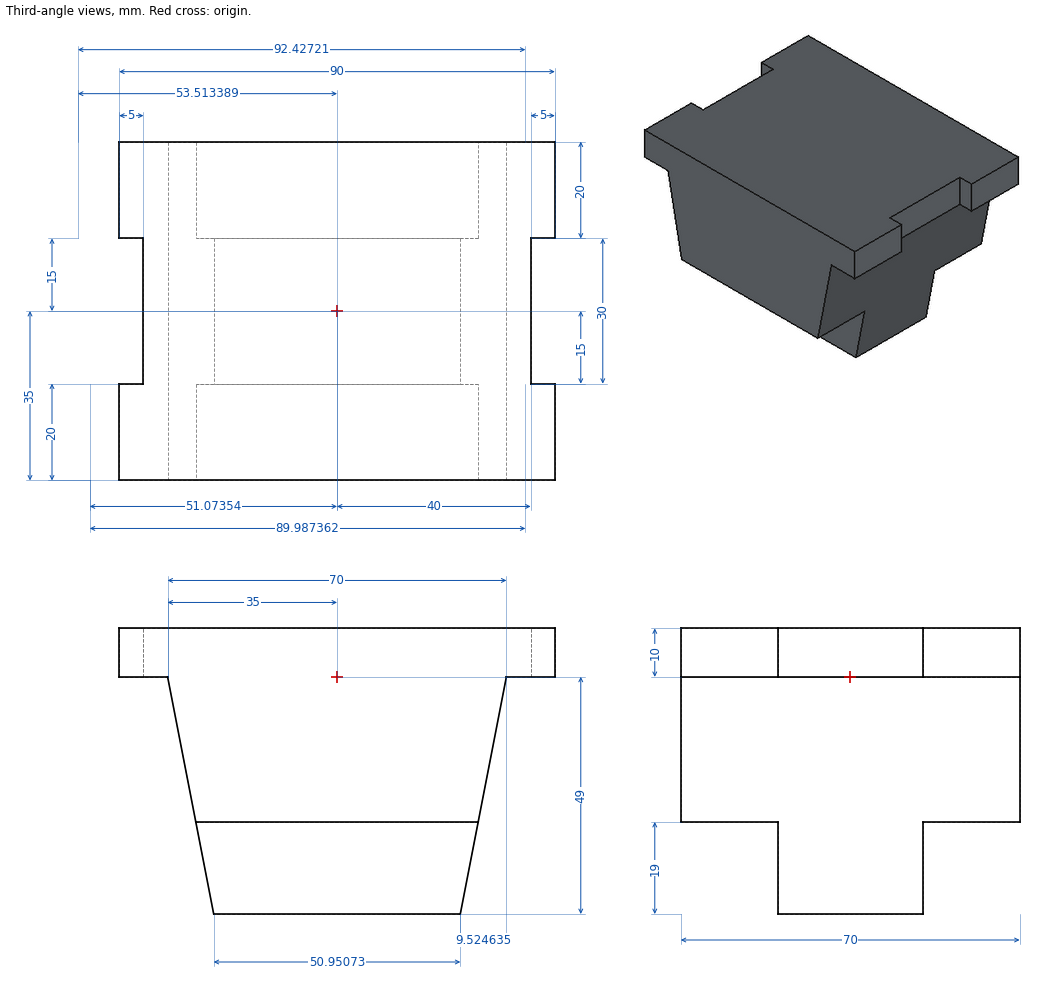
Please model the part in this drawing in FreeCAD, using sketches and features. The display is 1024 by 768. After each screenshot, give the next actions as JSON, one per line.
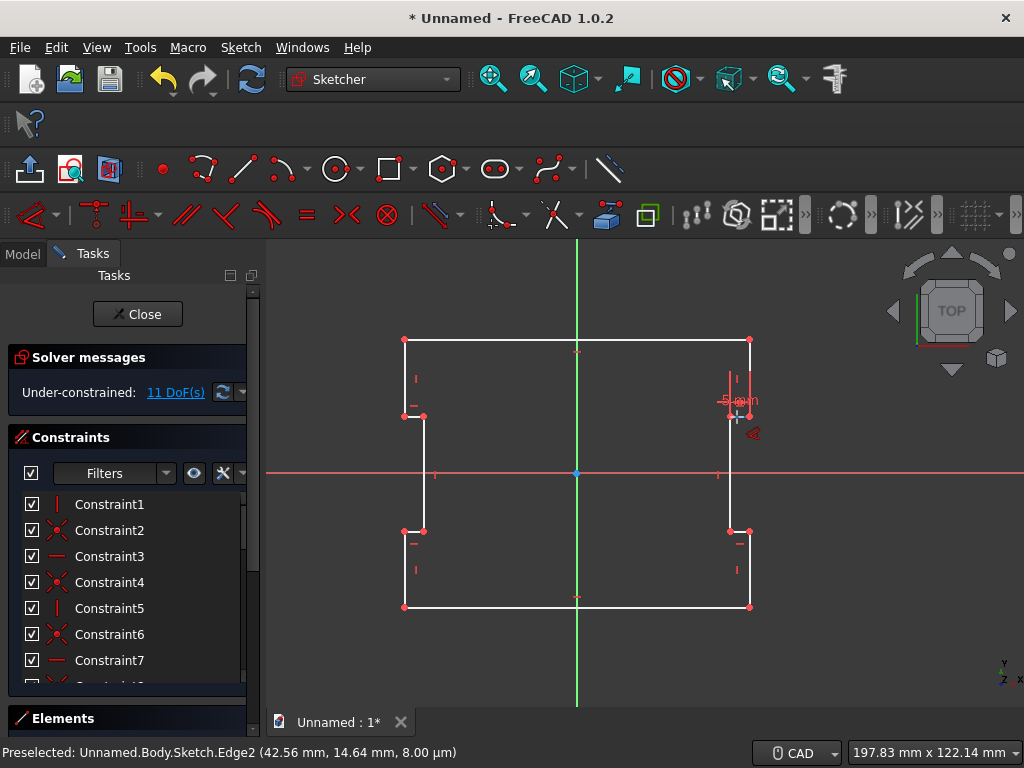
{"action": "scroll", "coordinate": [410, 417], "scroll_direction": "up", "scroll_amount": 5}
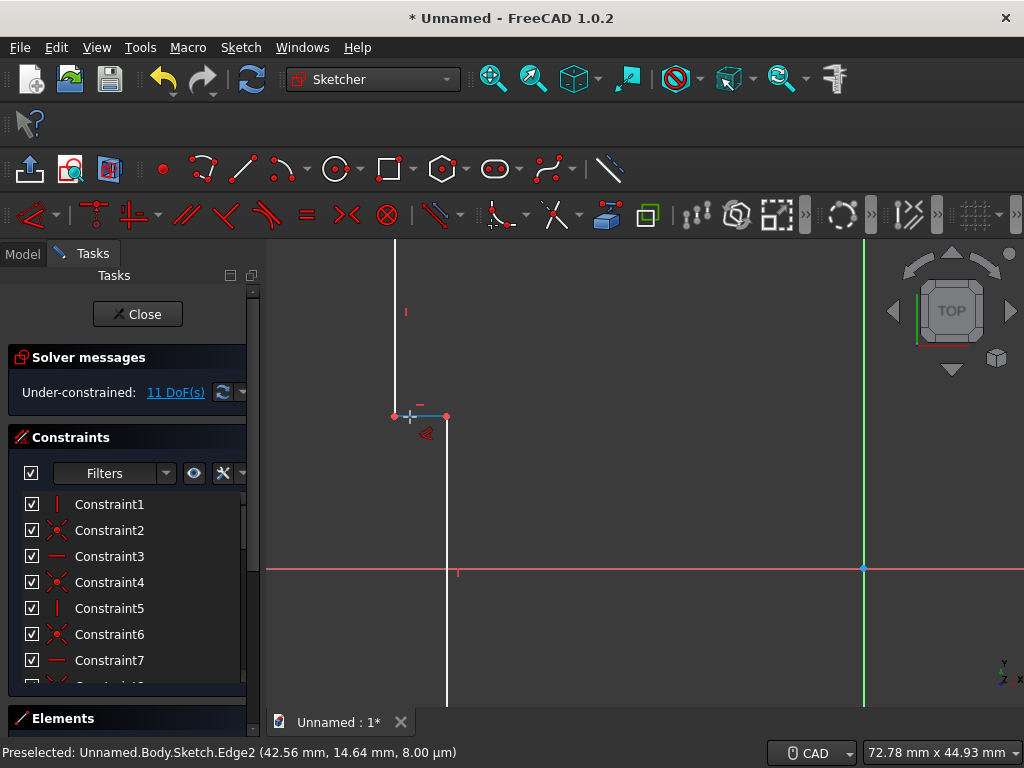
{"action": "left_click", "coordinate": [410, 416]}
{"action": "left_click", "coordinate": [421, 382]}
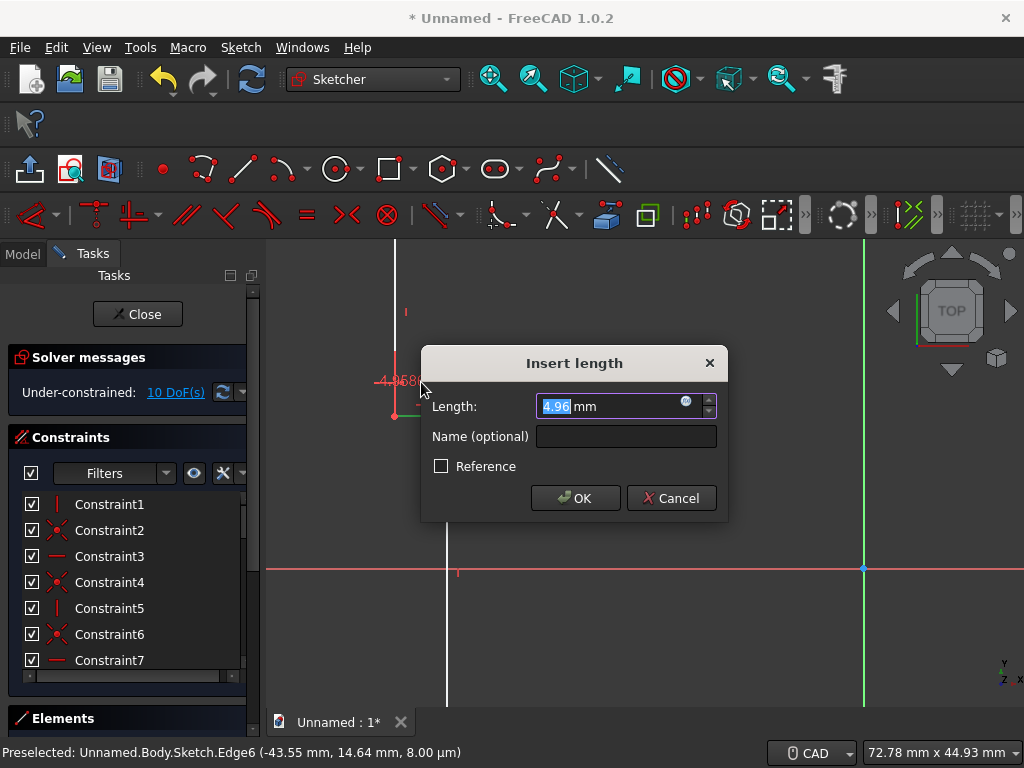
{"action": "type", "text": "5"}
{"action": "key", "text": "Return"}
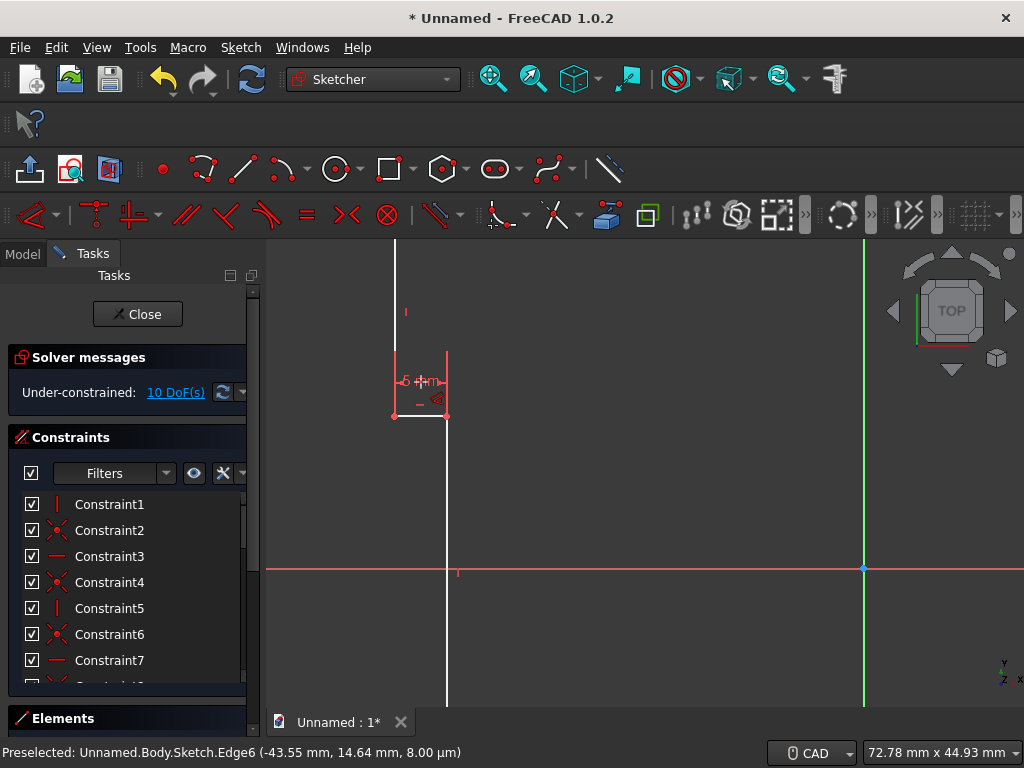
{"action": "scroll", "coordinate": [409, 417], "scroll_direction": "down", "scroll_amount": 5}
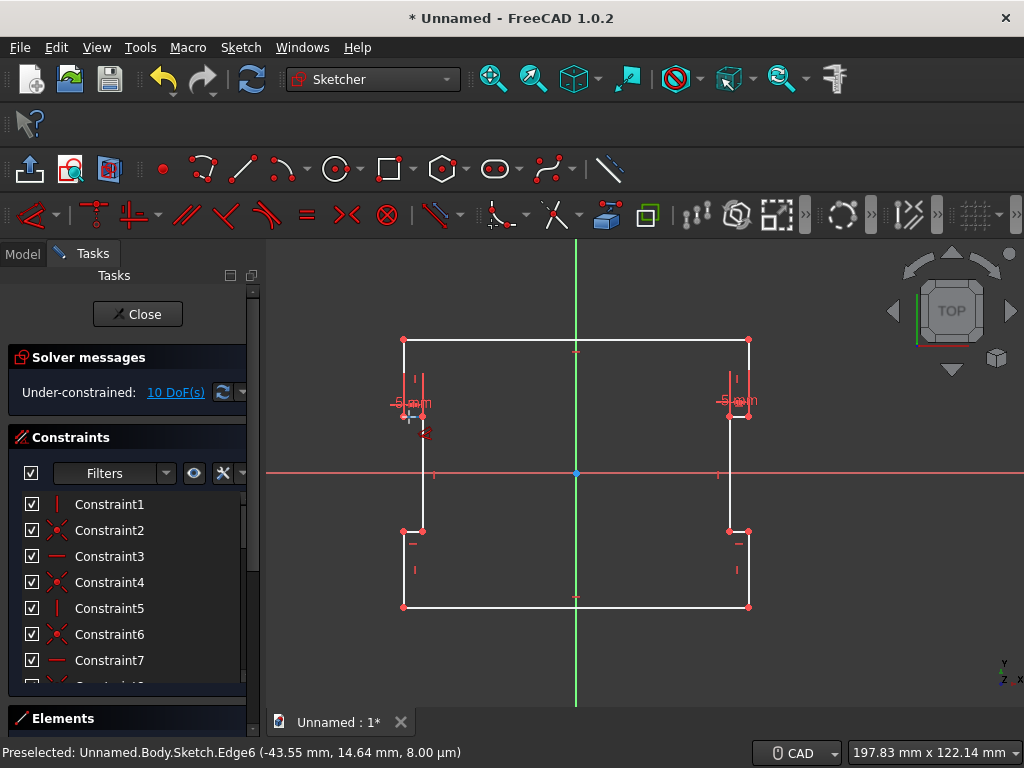
{"action": "scroll", "coordinate": [417, 532], "scroll_direction": "up", "scroll_amount": 5}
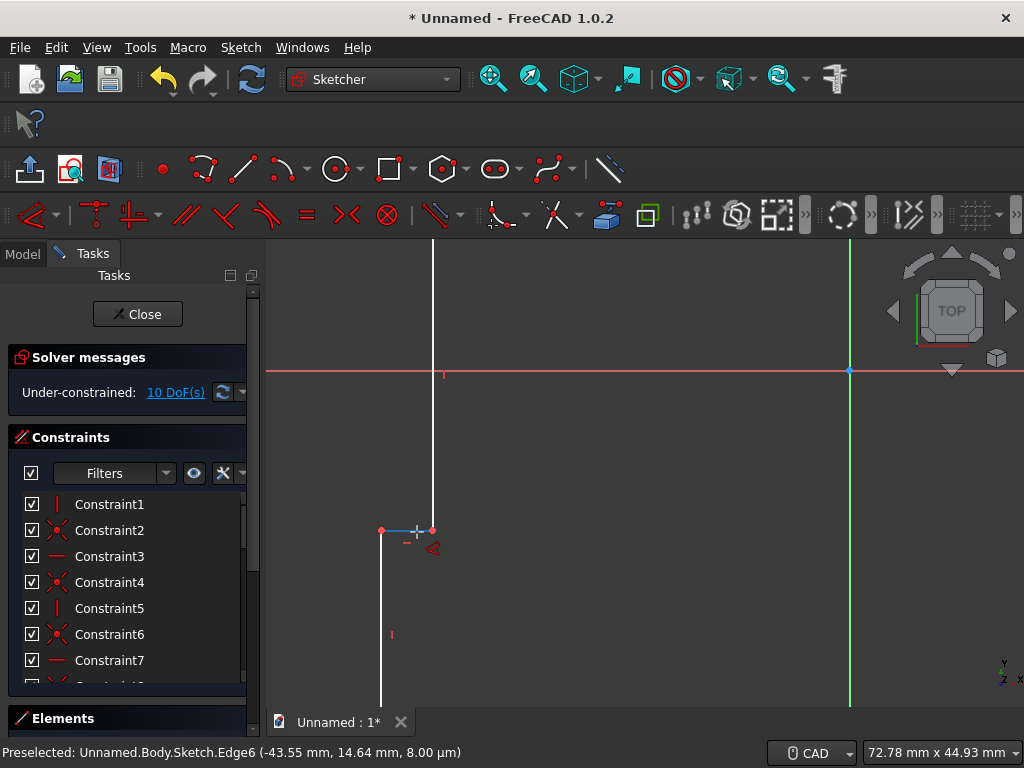
{"action": "left_click", "coordinate": [417, 531]}
{"action": "left_click", "coordinate": [407, 565]}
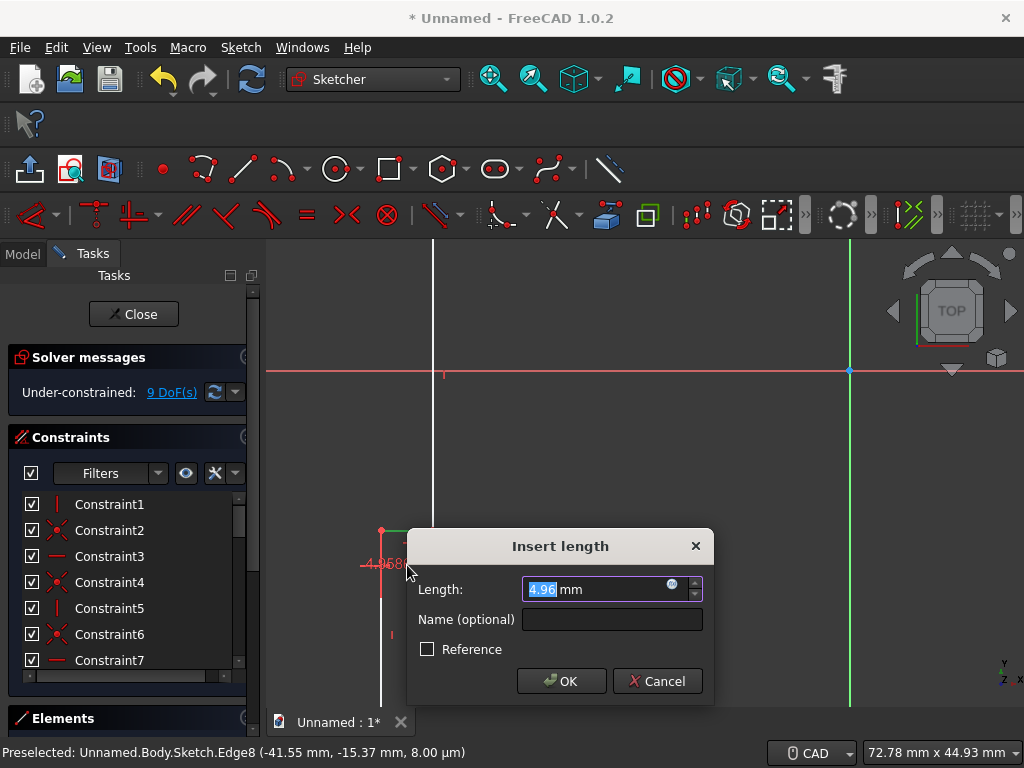
{"action": "type", "text": "5"}
{"action": "key", "text": "Return"}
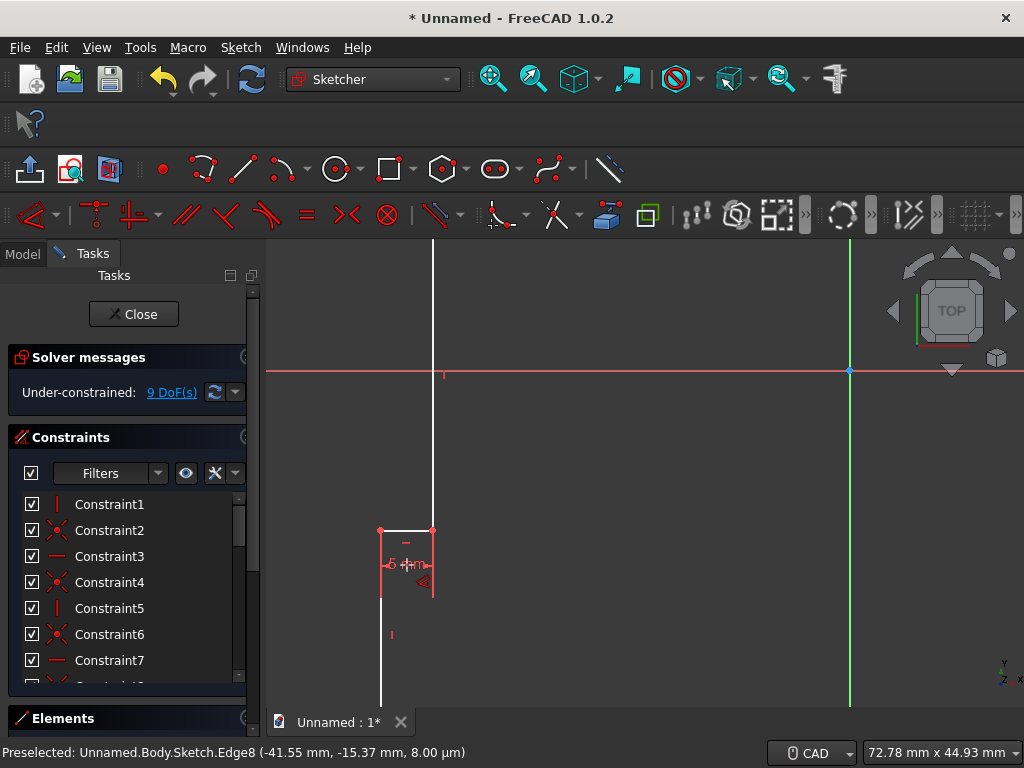
{"action": "scroll", "coordinate": [417, 532], "scroll_direction": "down", "scroll_amount": 5}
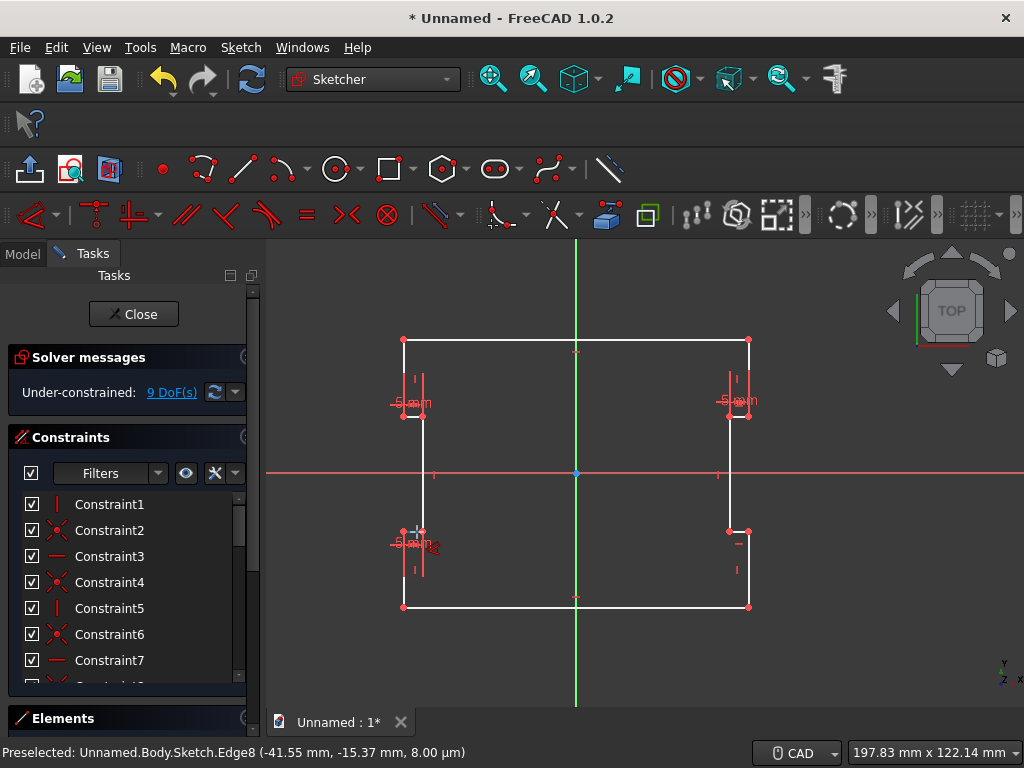
{"action": "scroll", "coordinate": [743, 532], "scroll_direction": "up", "scroll_amount": 5}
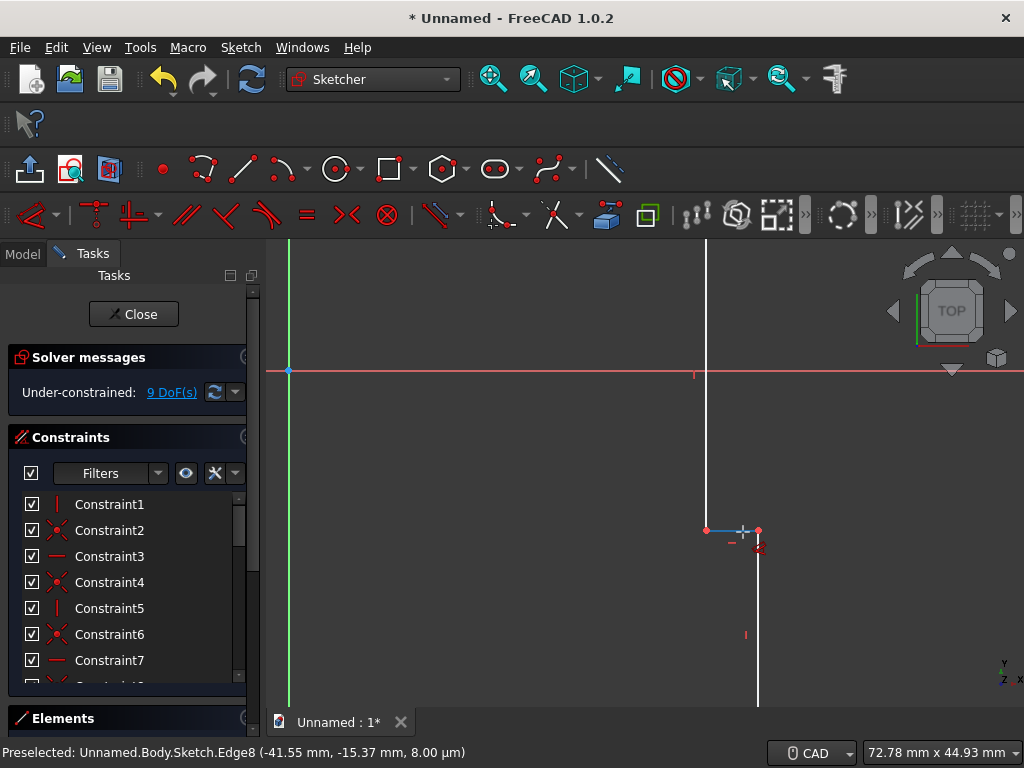
{"action": "left_click", "coordinate": [742, 531]}
{"action": "left_click", "coordinate": [732, 565]}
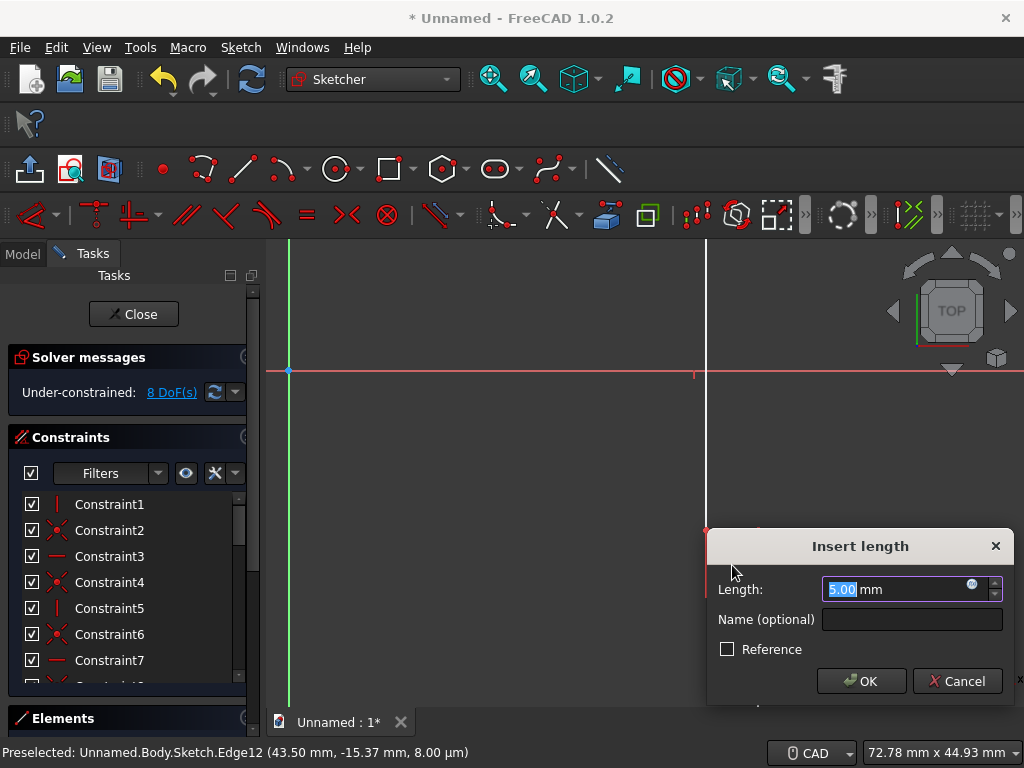
{"action": "type", "text": "5"}
{"action": "key", "text": "Return"}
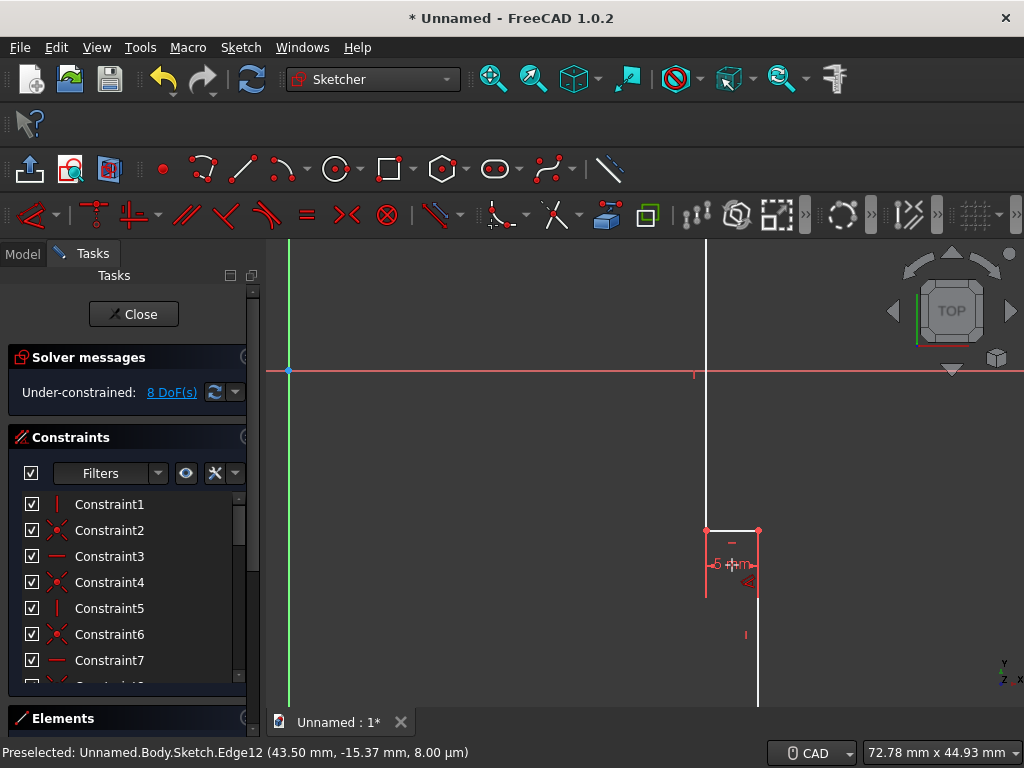
{"action": "left_click", "coordinate": [706, 437]}
{"action": "left_click", "coordinate": [740, 399]}